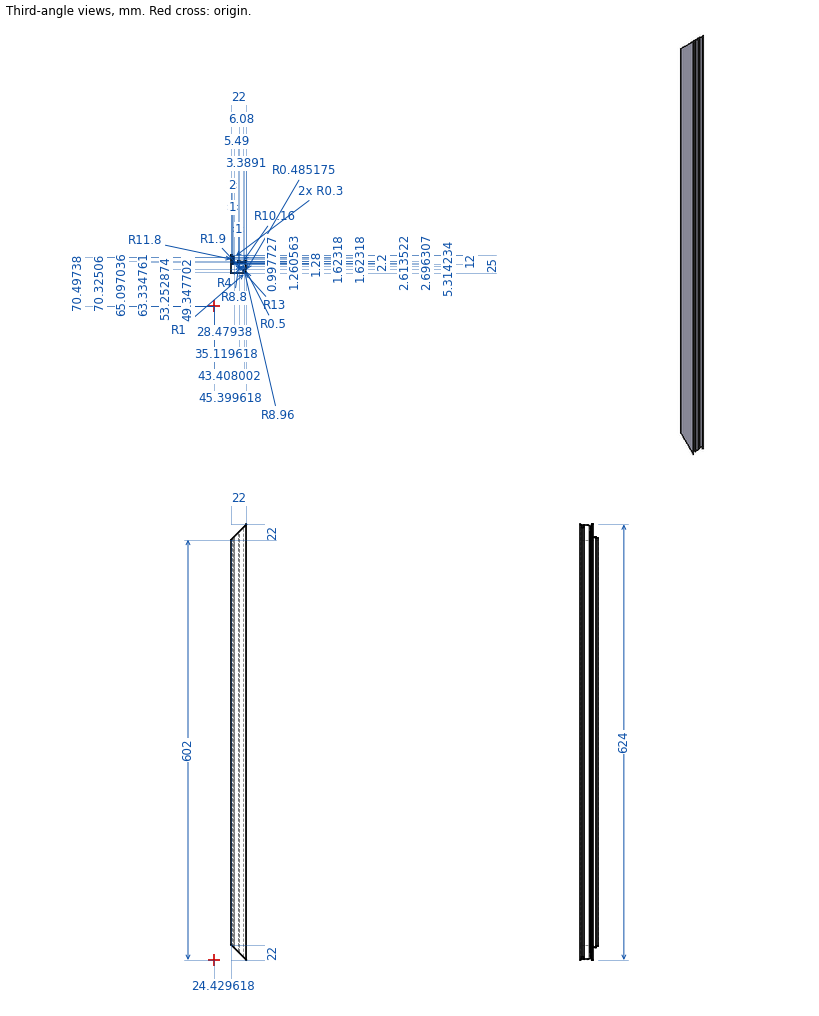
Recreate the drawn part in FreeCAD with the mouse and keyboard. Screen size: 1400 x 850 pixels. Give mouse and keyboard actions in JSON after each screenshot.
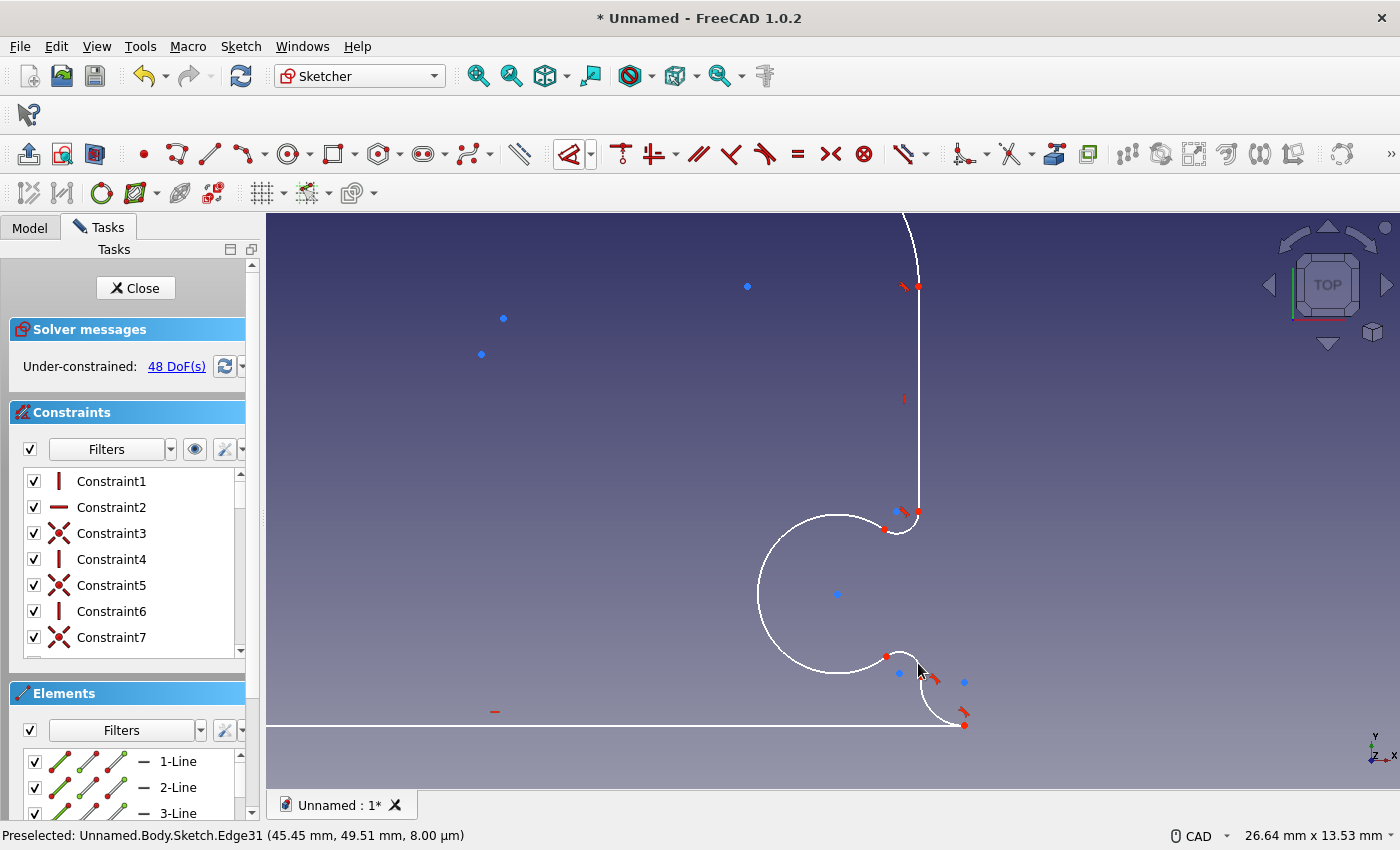
{"action": "left_click", "coordinate": [918, 662]}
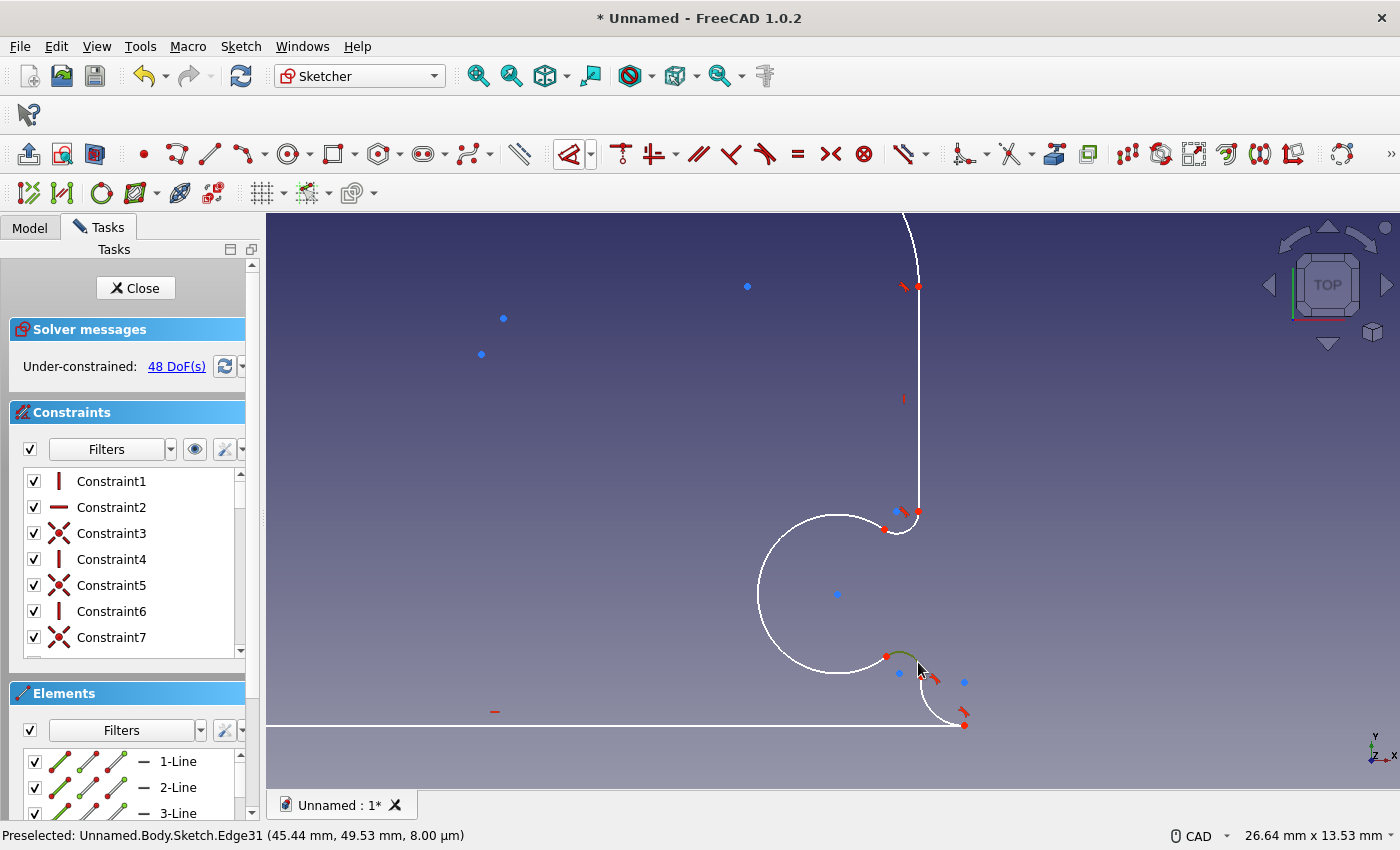
{"action": "left_click", "coordinate": [786, 533]}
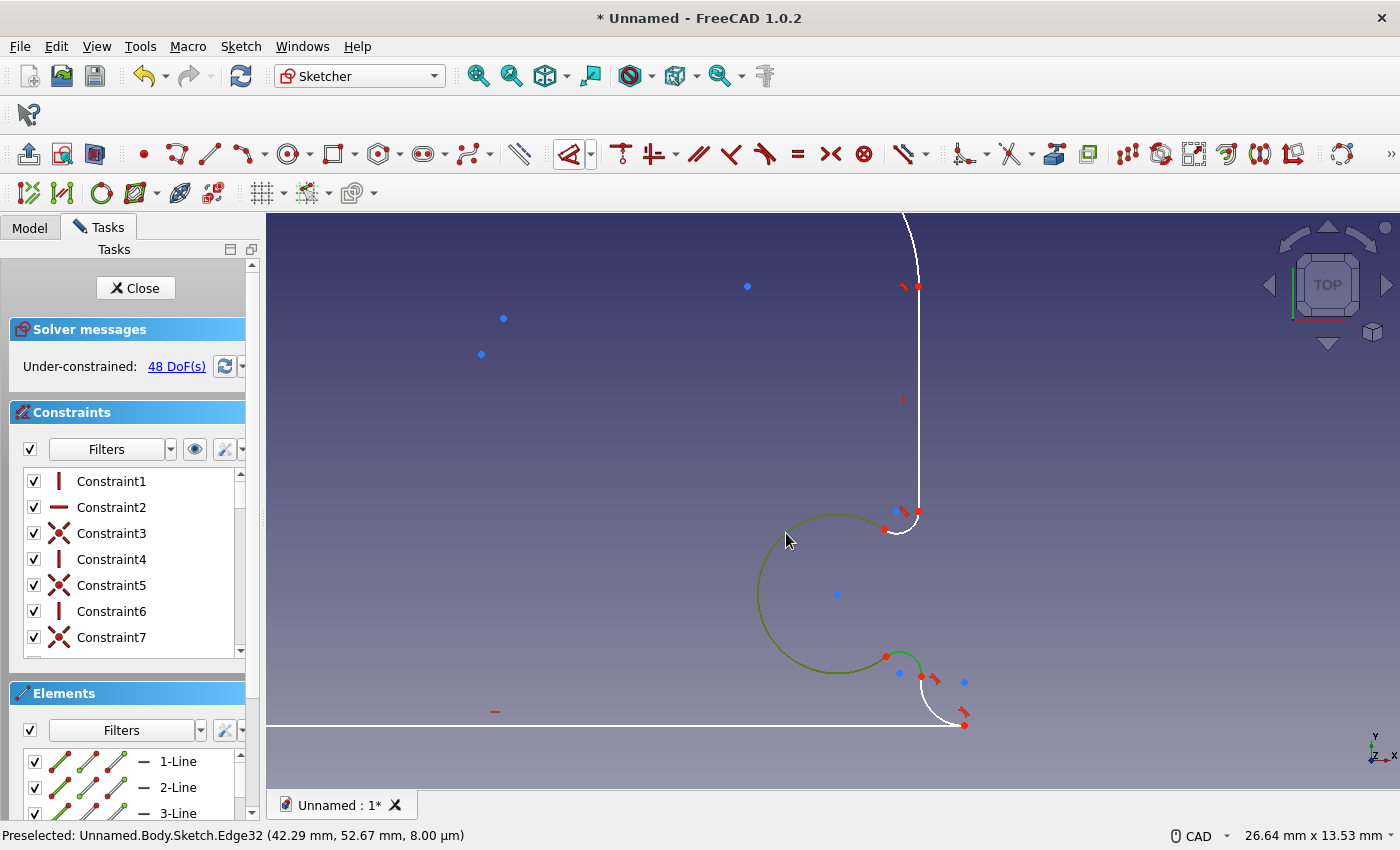
{"action": "key", "text": "t"}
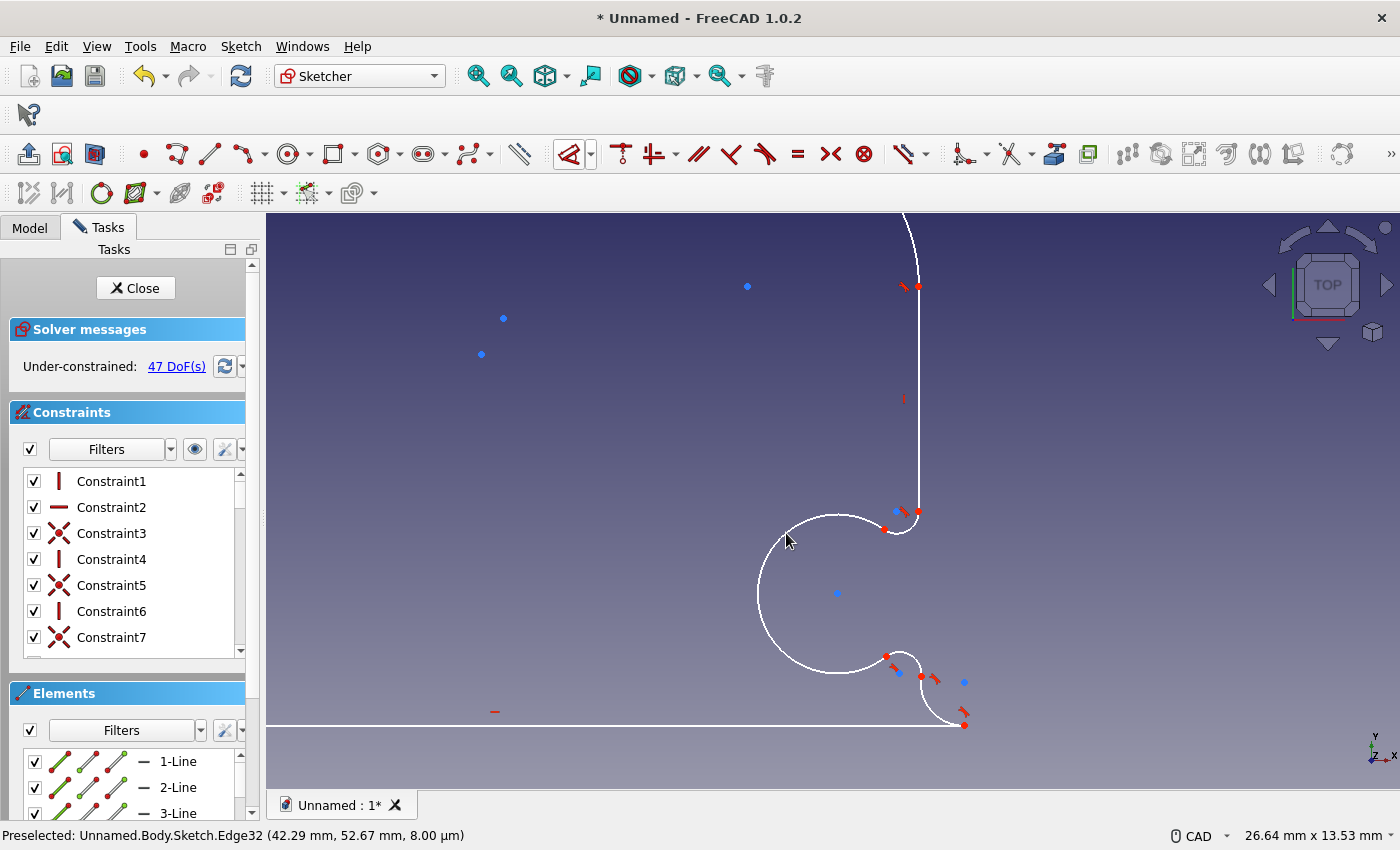
{"action": "left_click", "coordinate": [786, 533]}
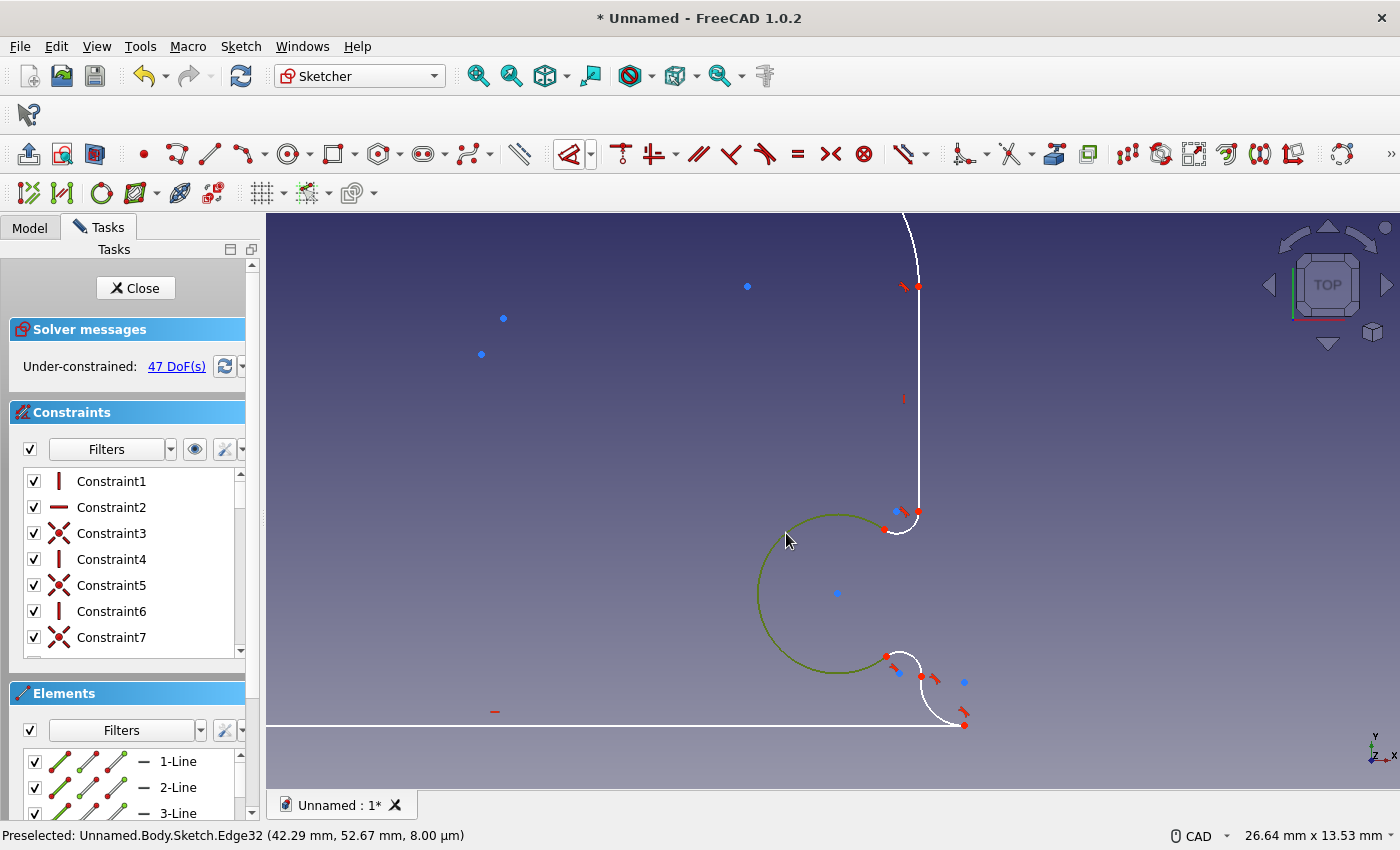
{"action": "left_click", "coordinate": [898, 534]}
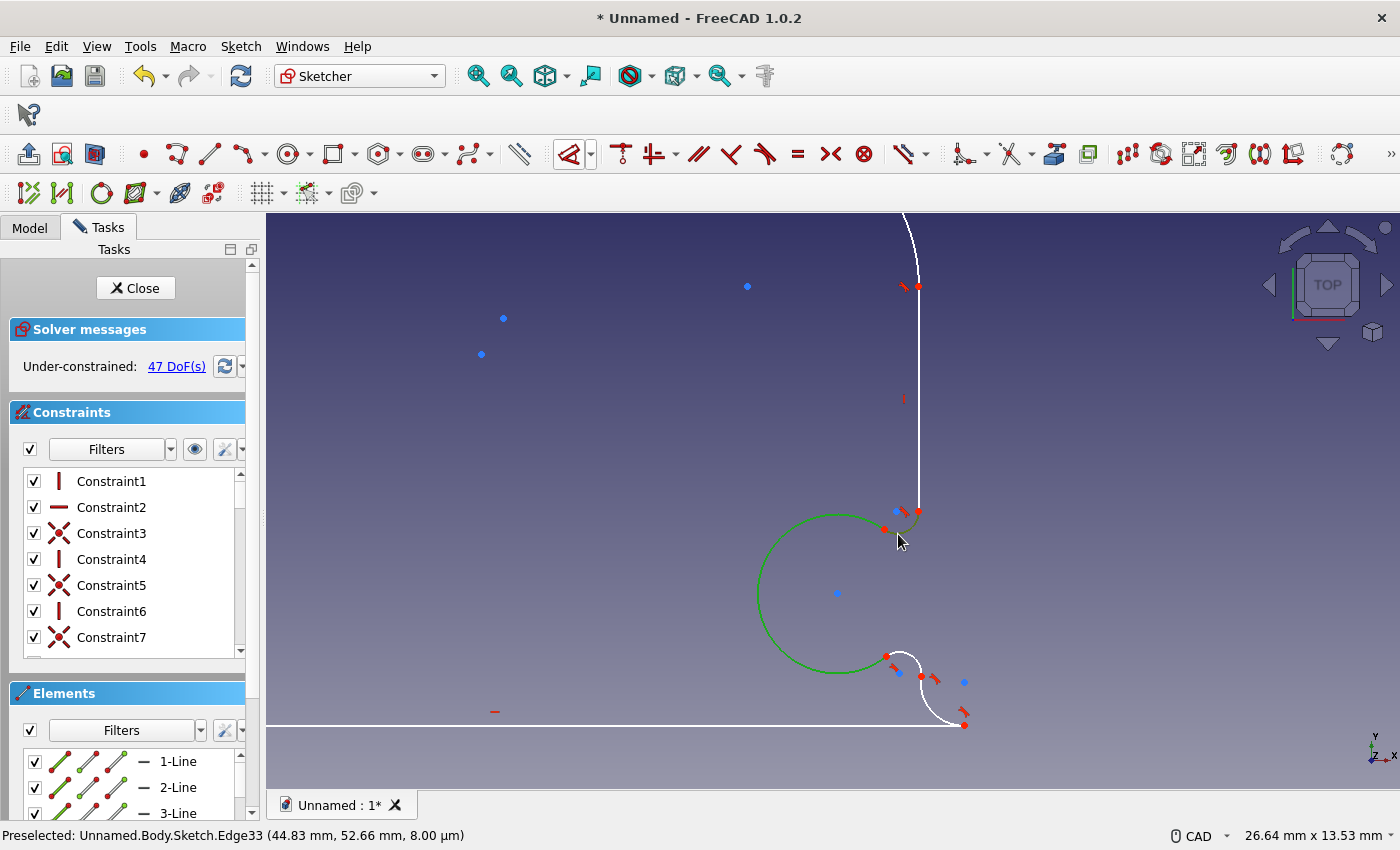
{"action": "left_click", "coordinate": [765, 154]}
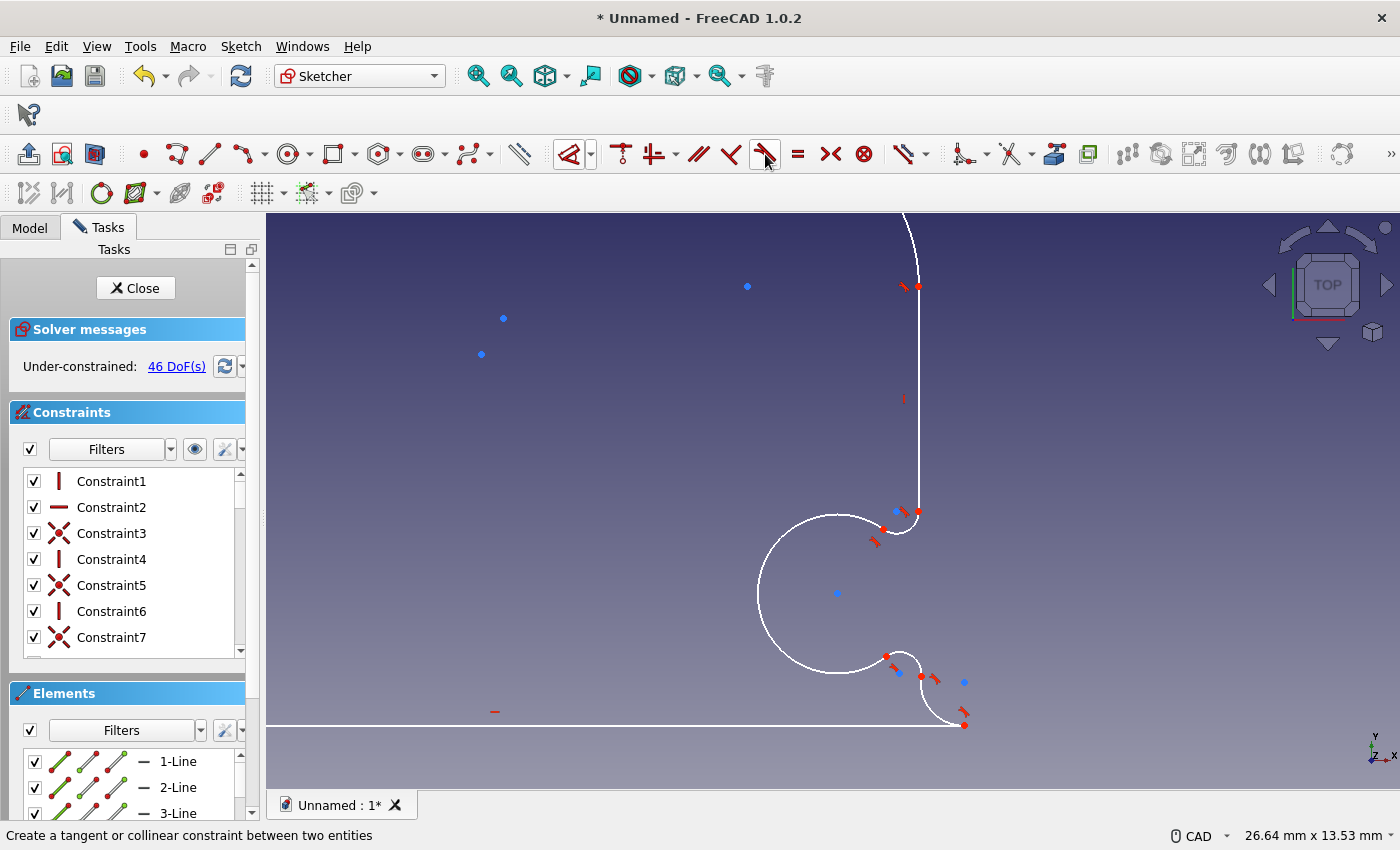
{"action": "scroll", "coordinate": [922, 681], "scroll_direction": "down", "scroll_amount": 5}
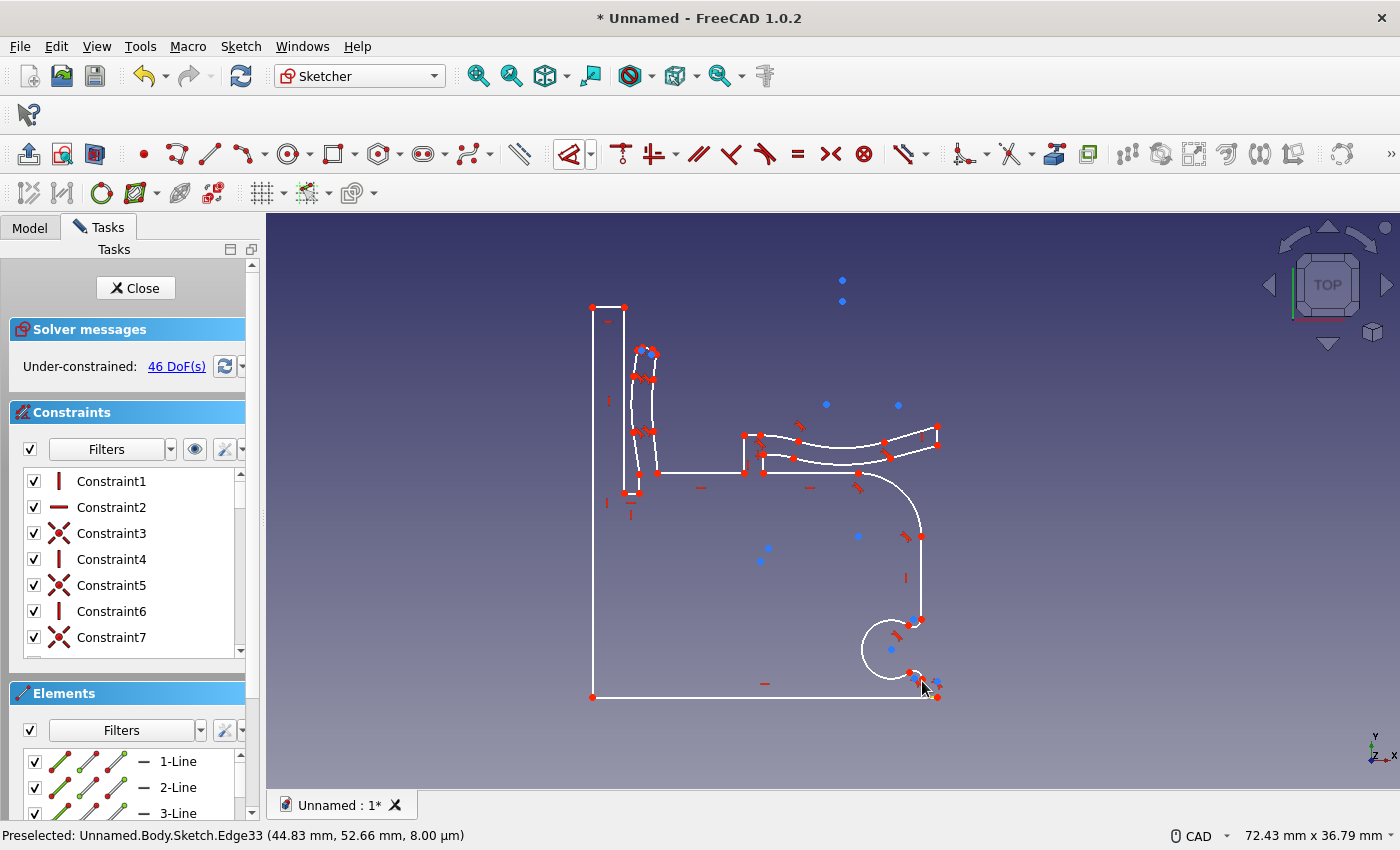
{"action": "scroll", "coordinate": [822, 464], "scroll_direction": "up", "scroll_amount": 2}